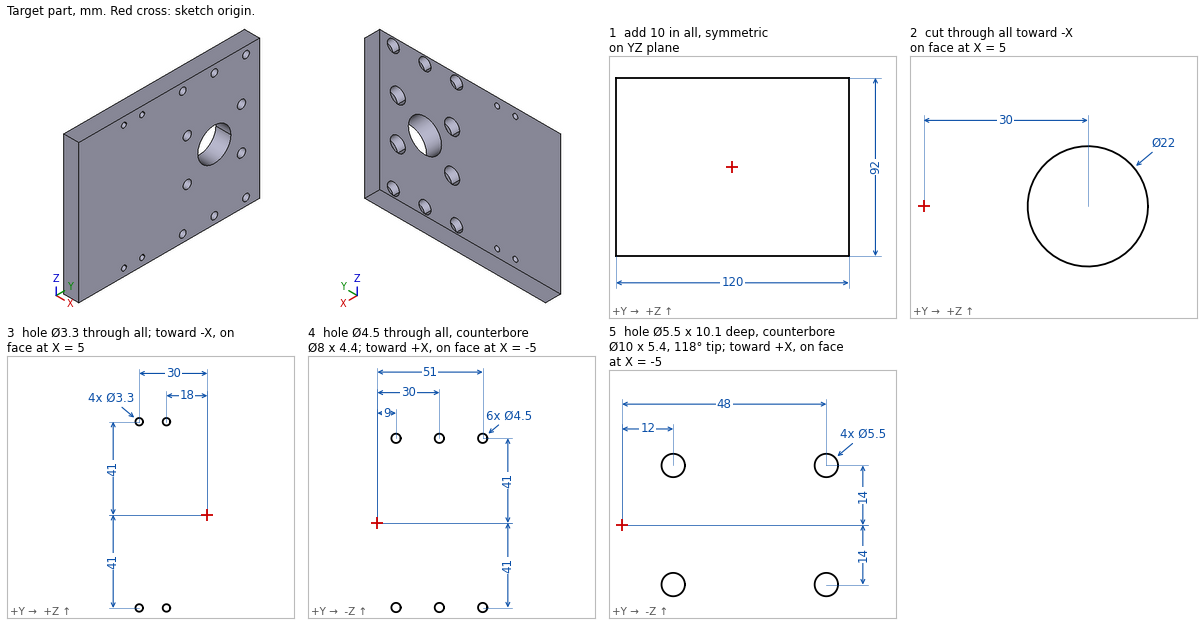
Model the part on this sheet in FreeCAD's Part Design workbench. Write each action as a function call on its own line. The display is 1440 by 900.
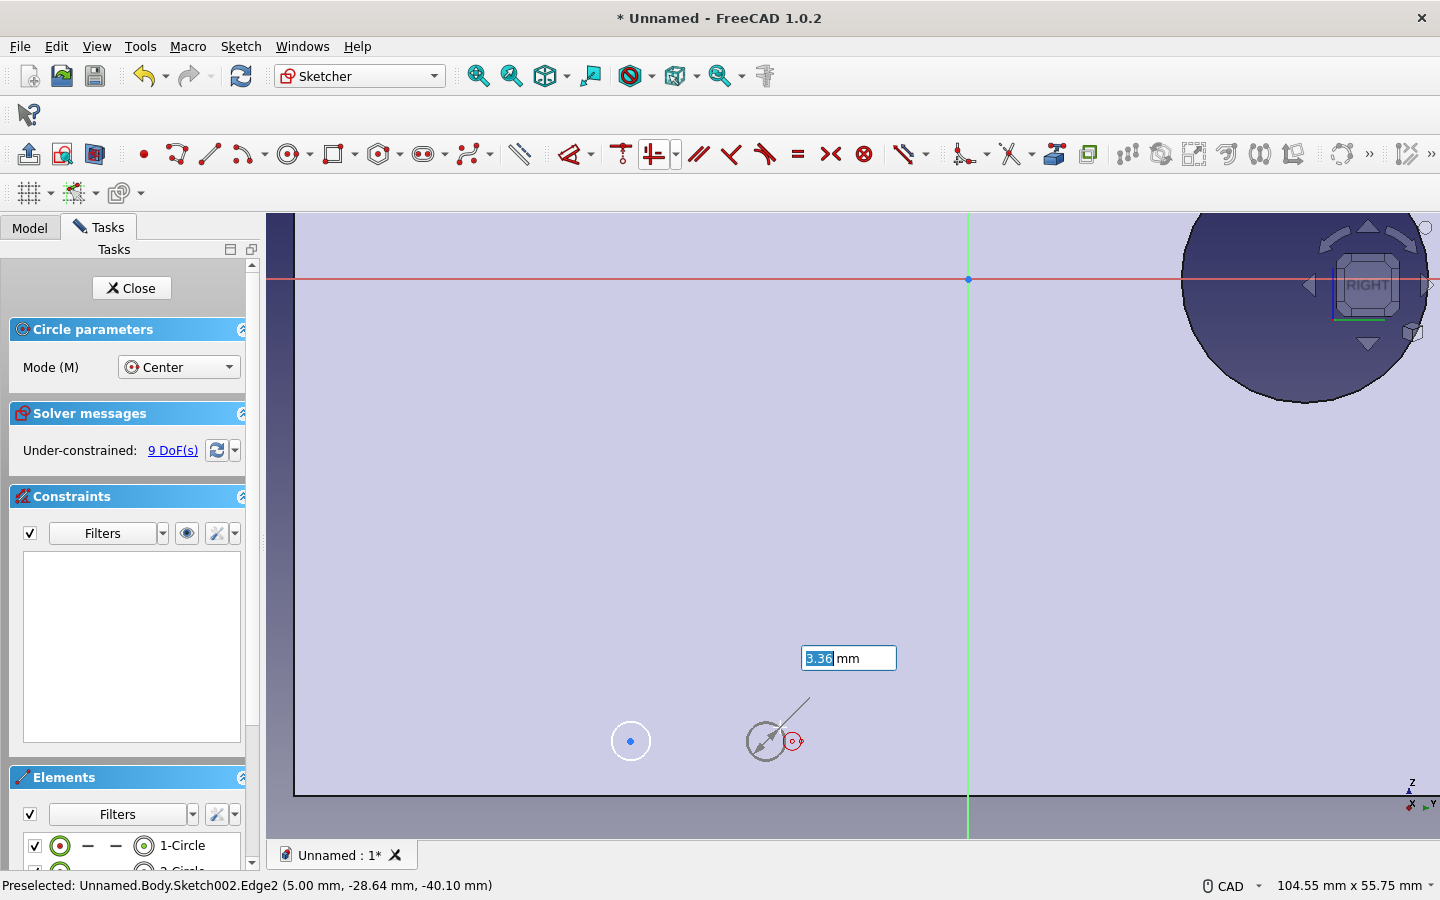
click(779, 727)
key(Escape)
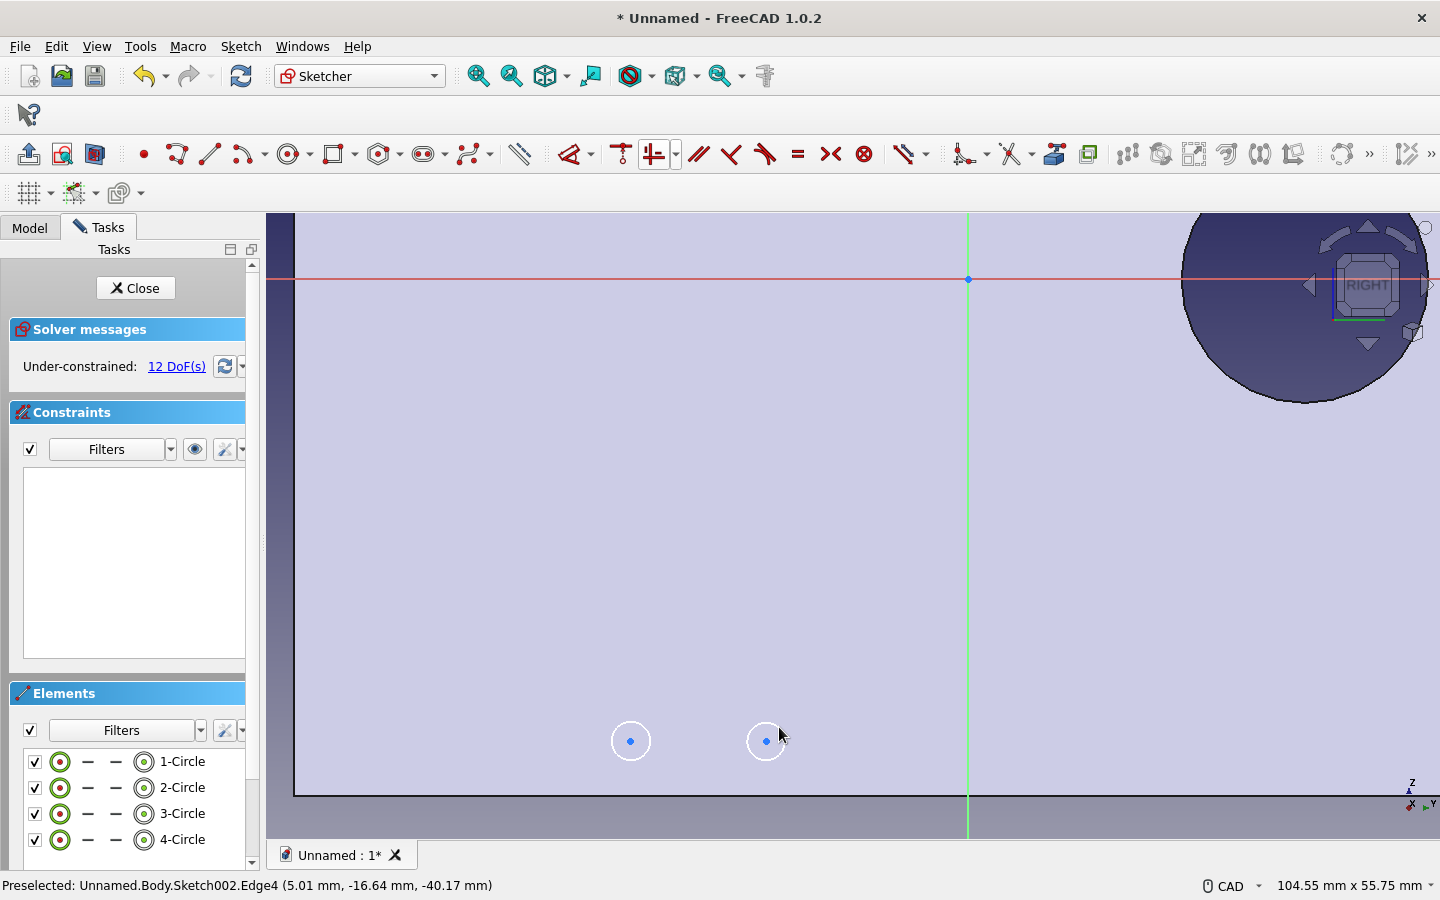
scroll(780, 727, down, 4)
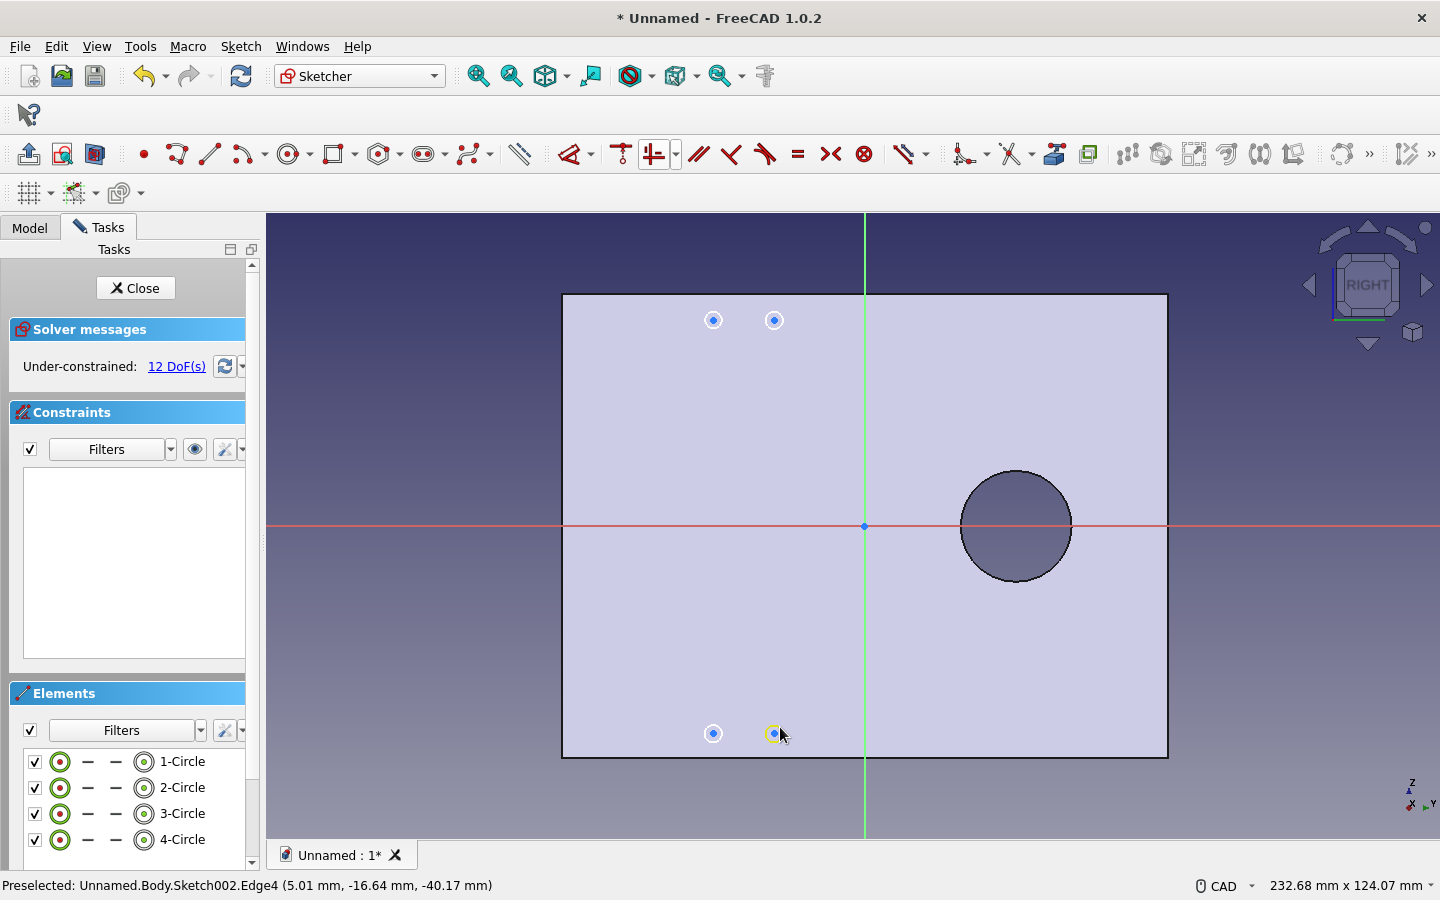
scroll(719, 314, up, 3)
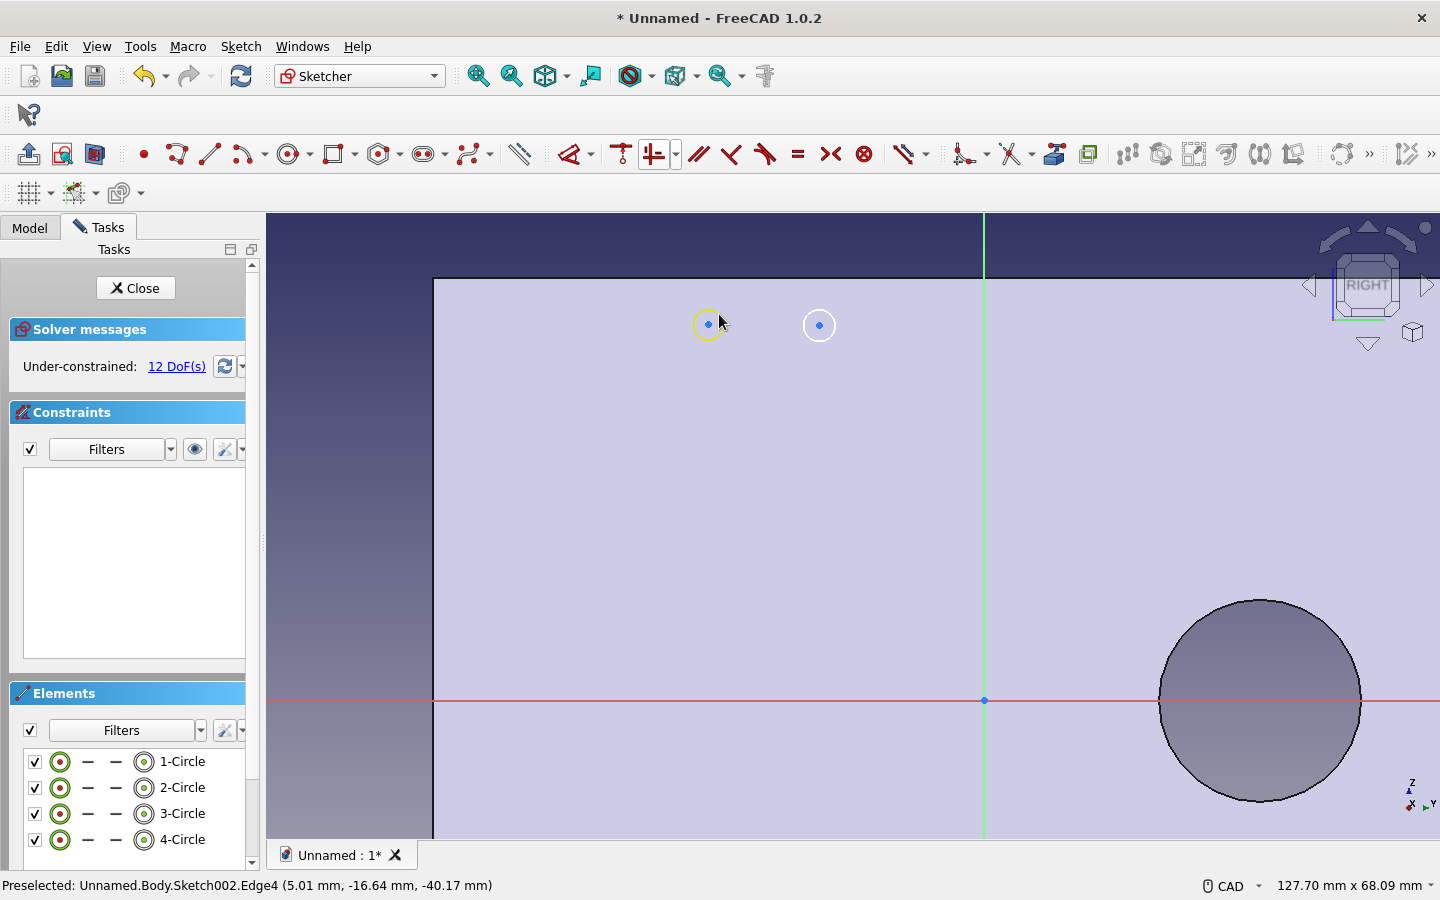
click(719, 314)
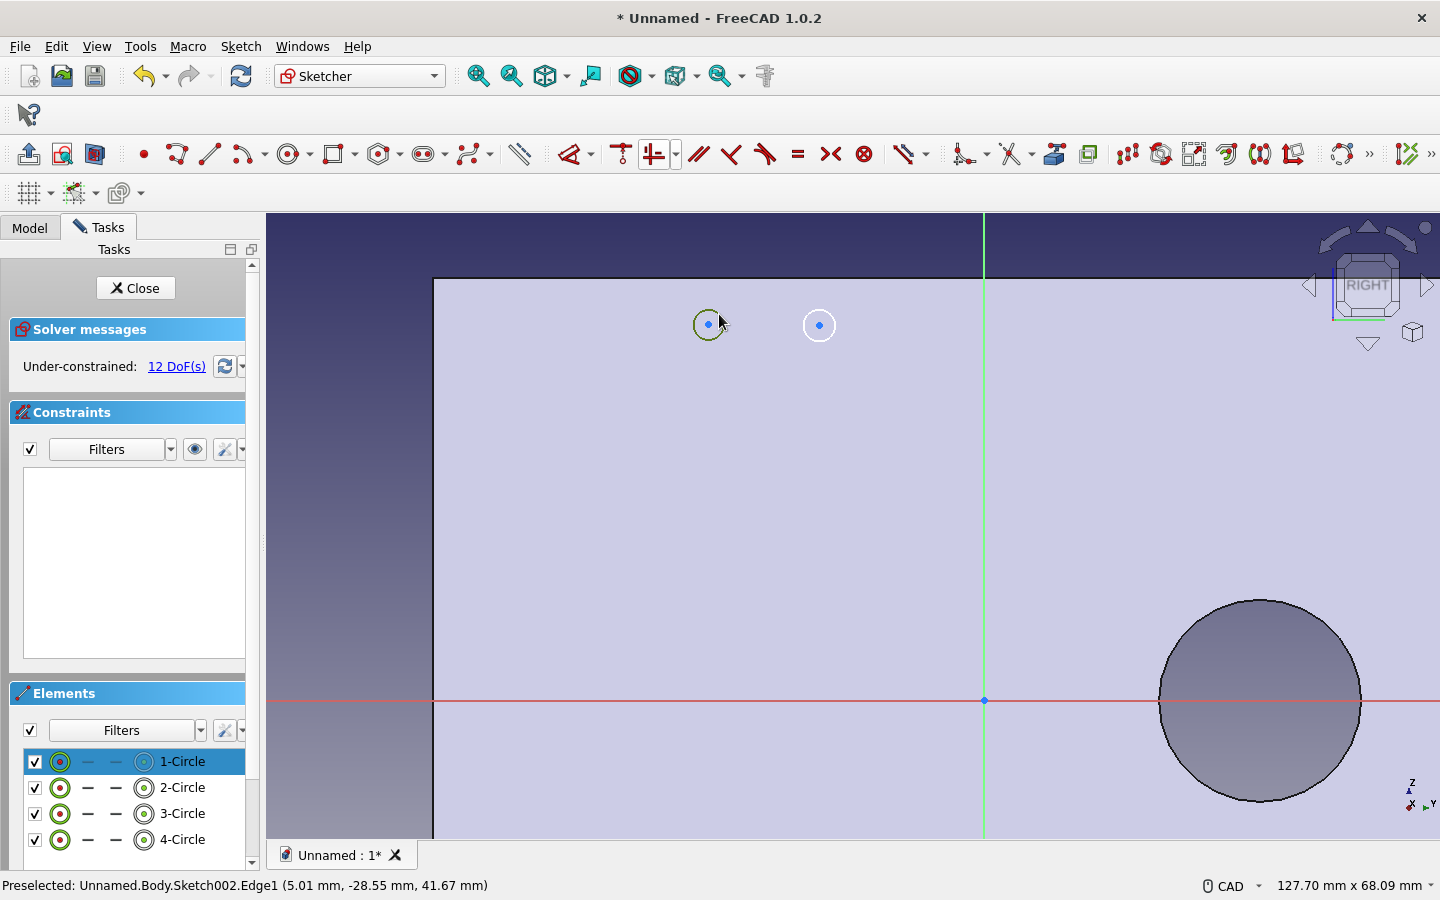
click(830, 314)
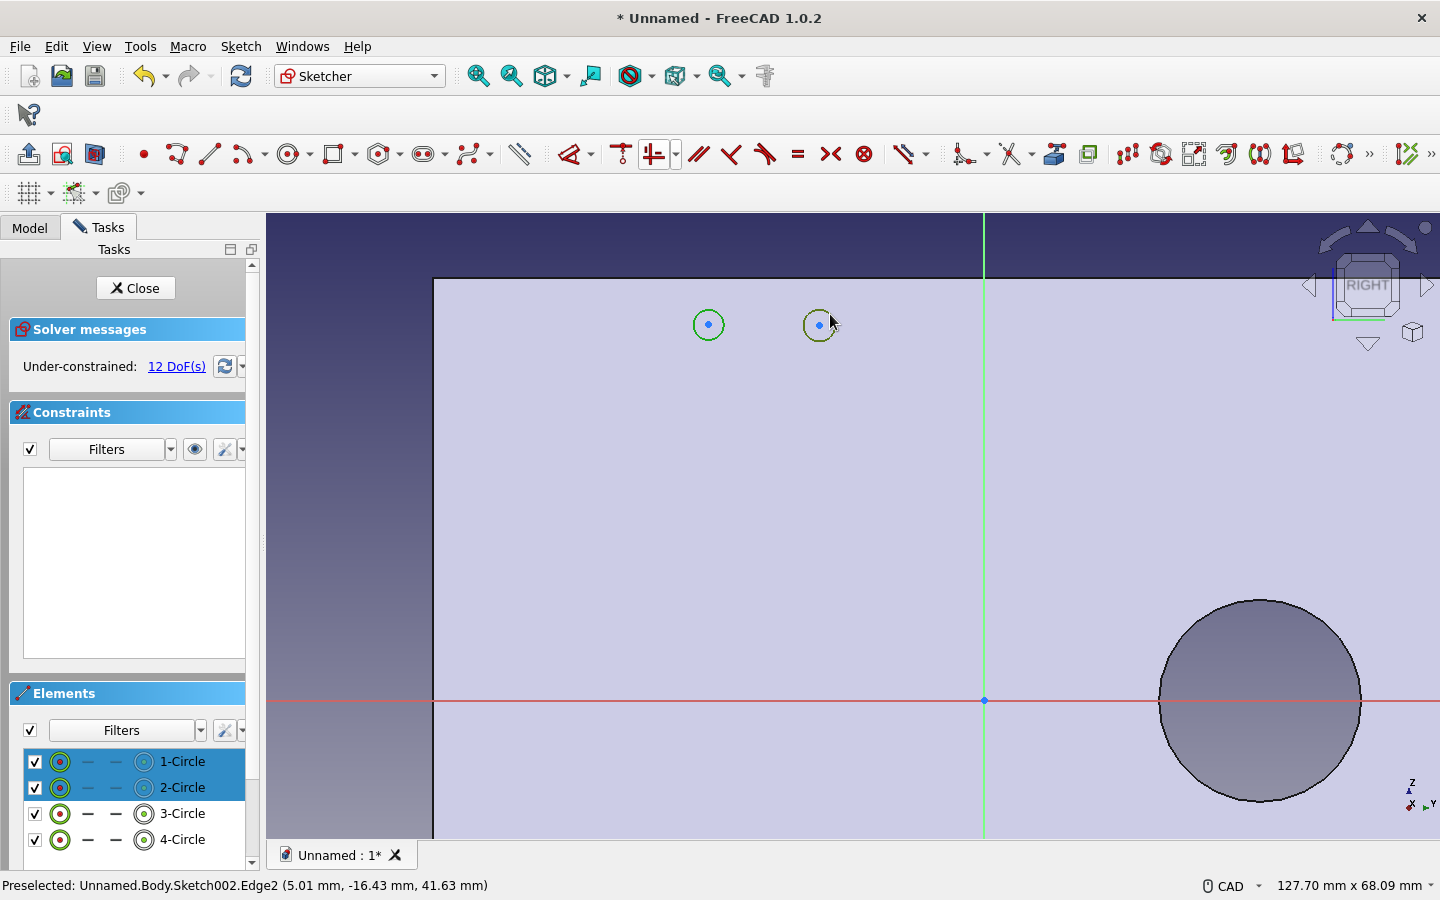
scroll(718, 313, down, 3)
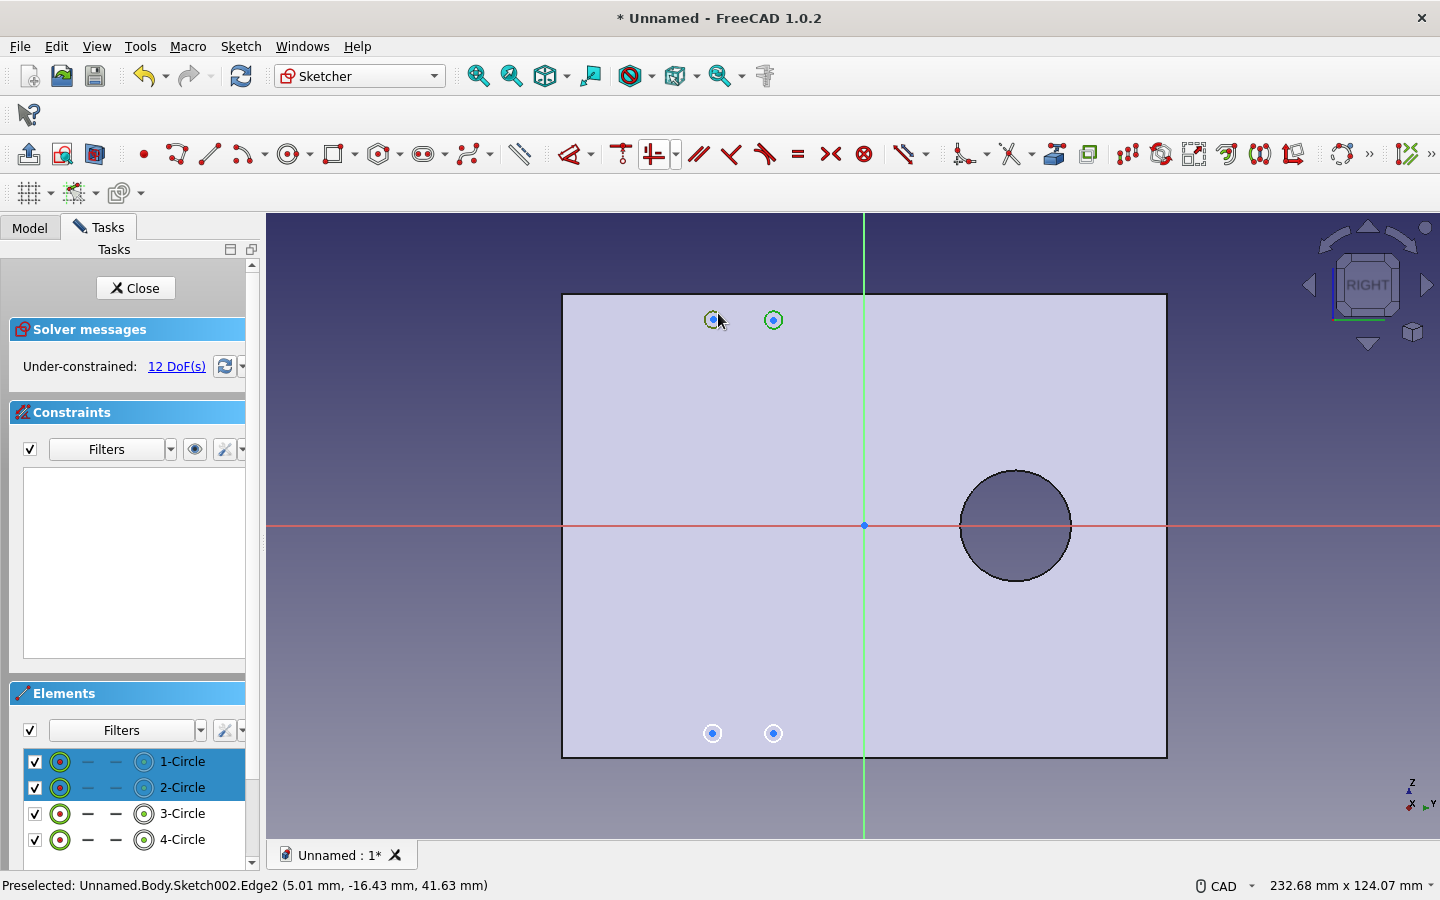
scroll(719, 727, up, 3)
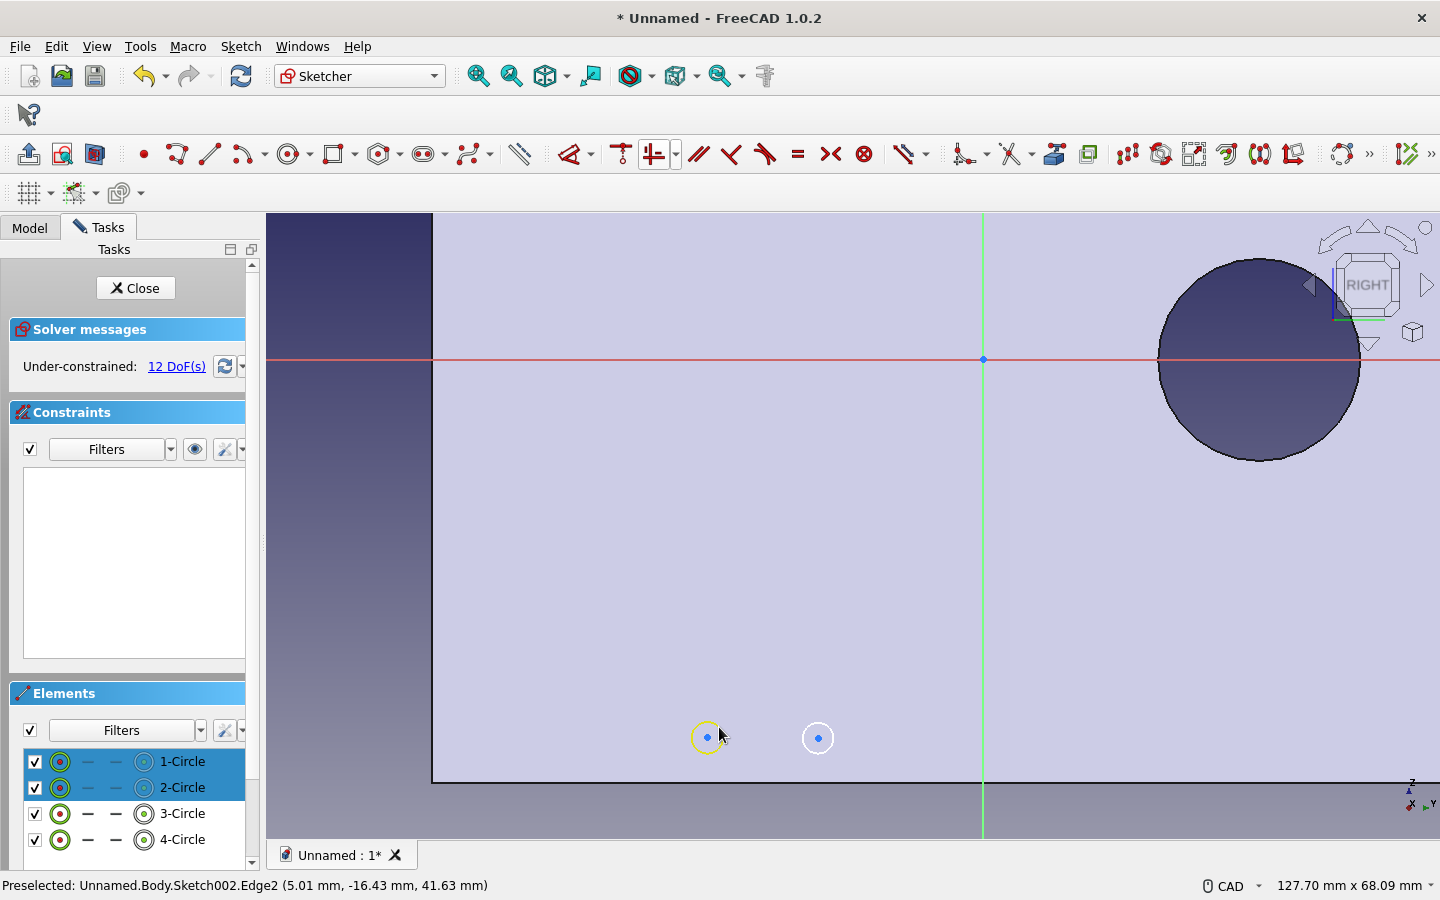
click(718, 727)